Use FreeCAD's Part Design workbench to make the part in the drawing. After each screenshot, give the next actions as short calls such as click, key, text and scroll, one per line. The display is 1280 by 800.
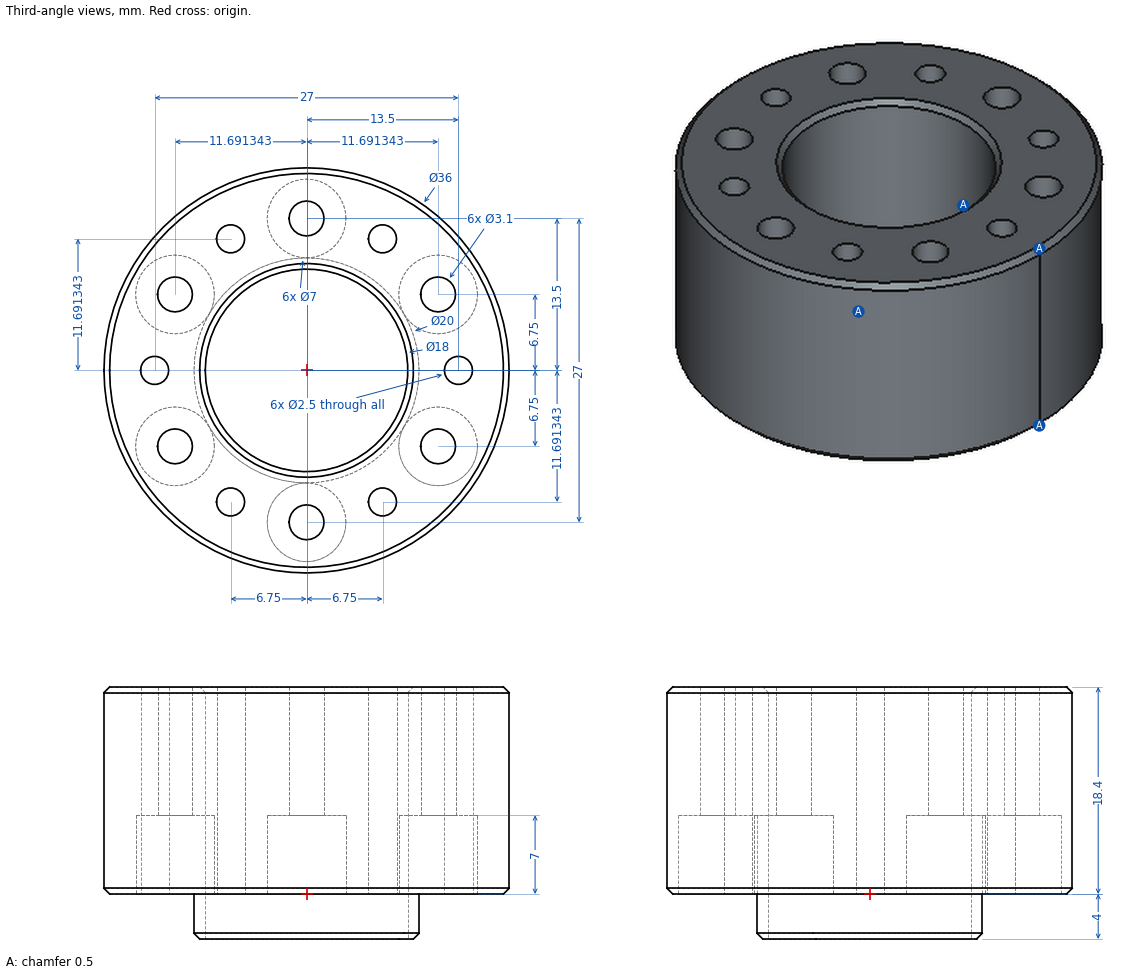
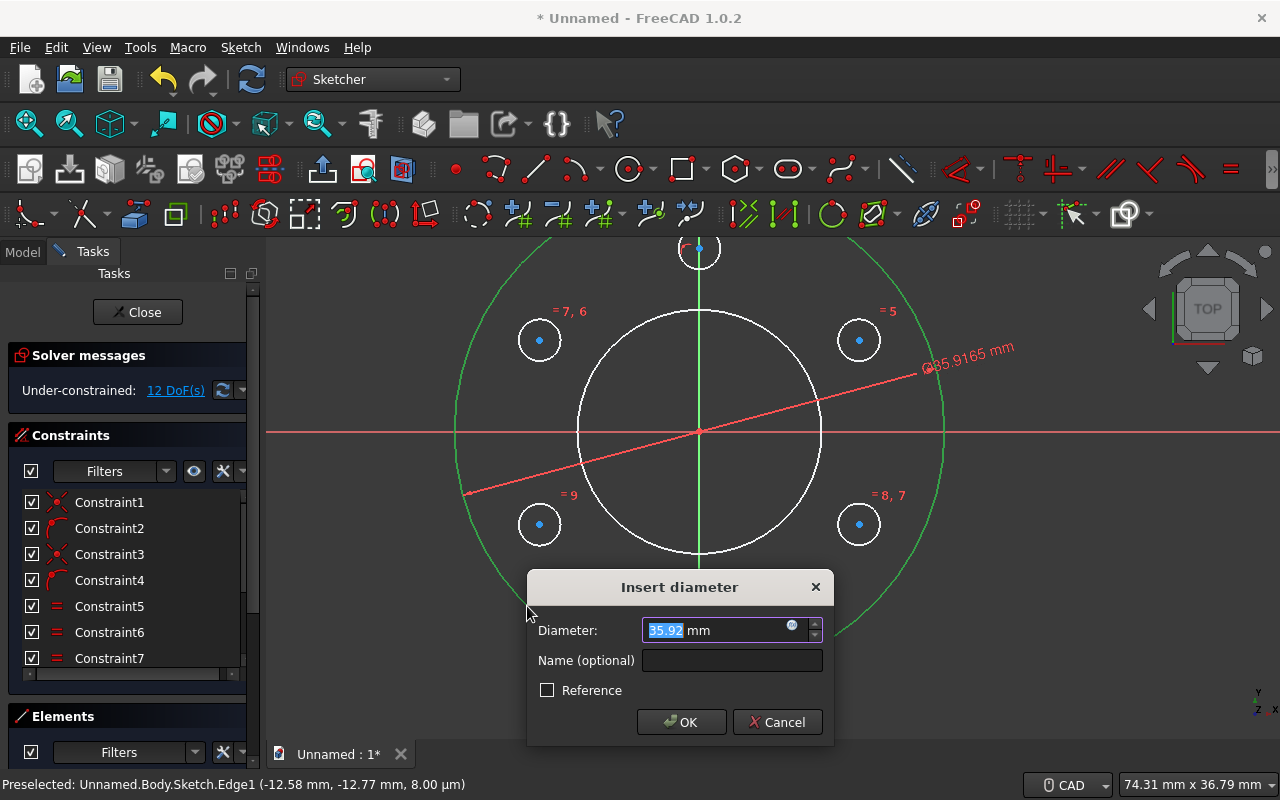
text(36)
key(Return)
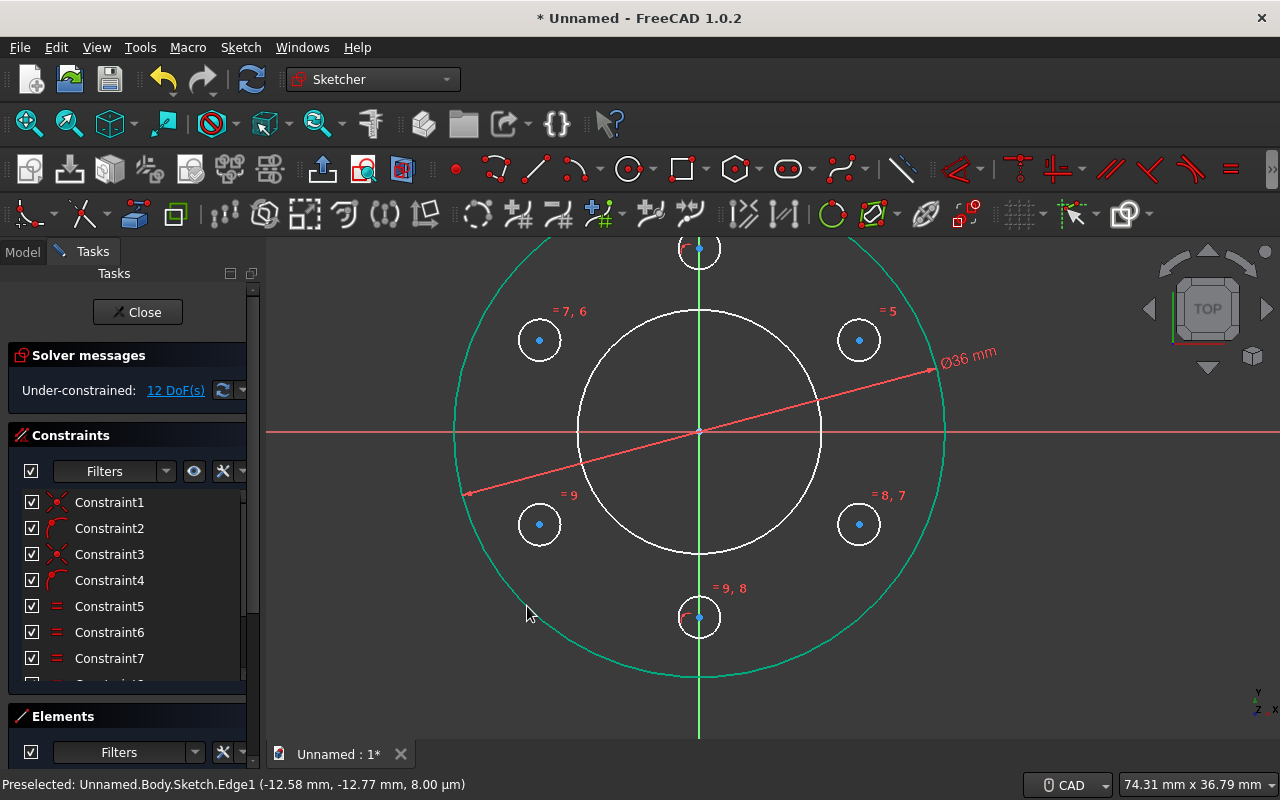
click(874, 325)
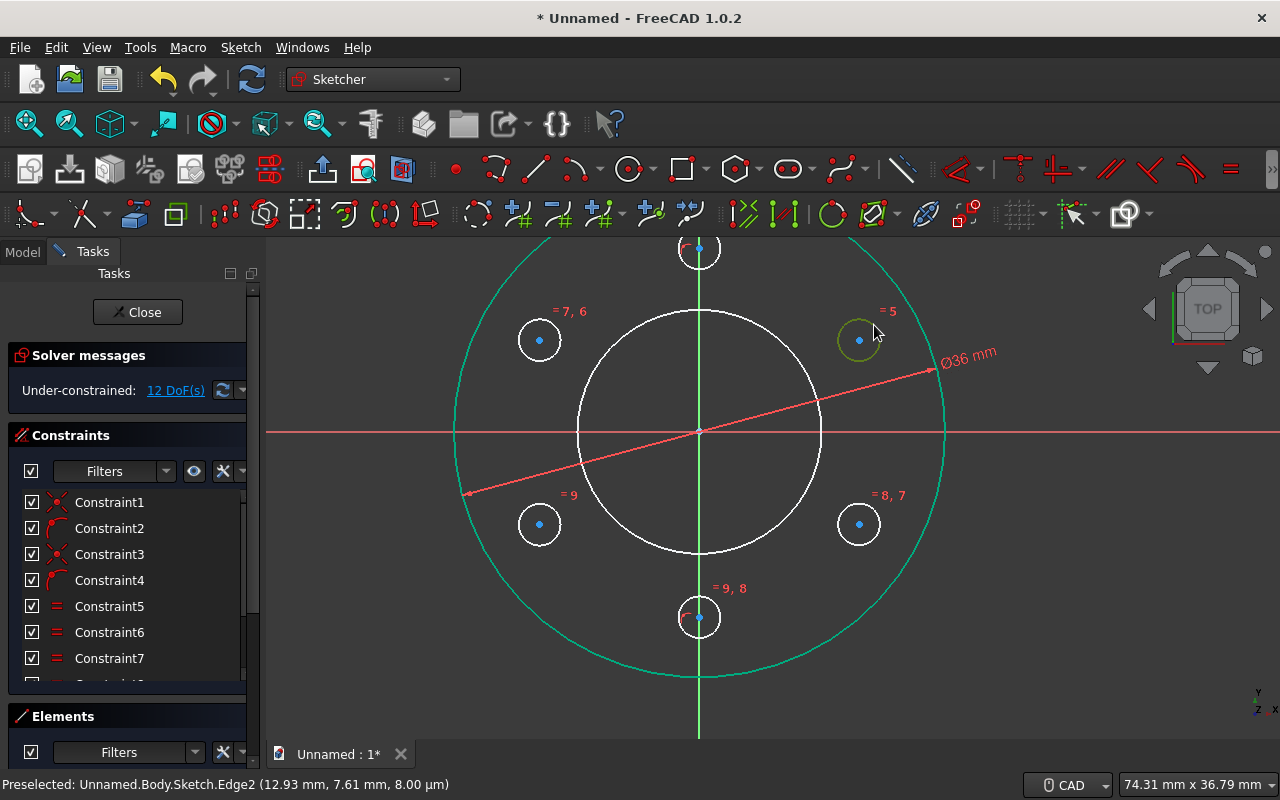
click(982, 170)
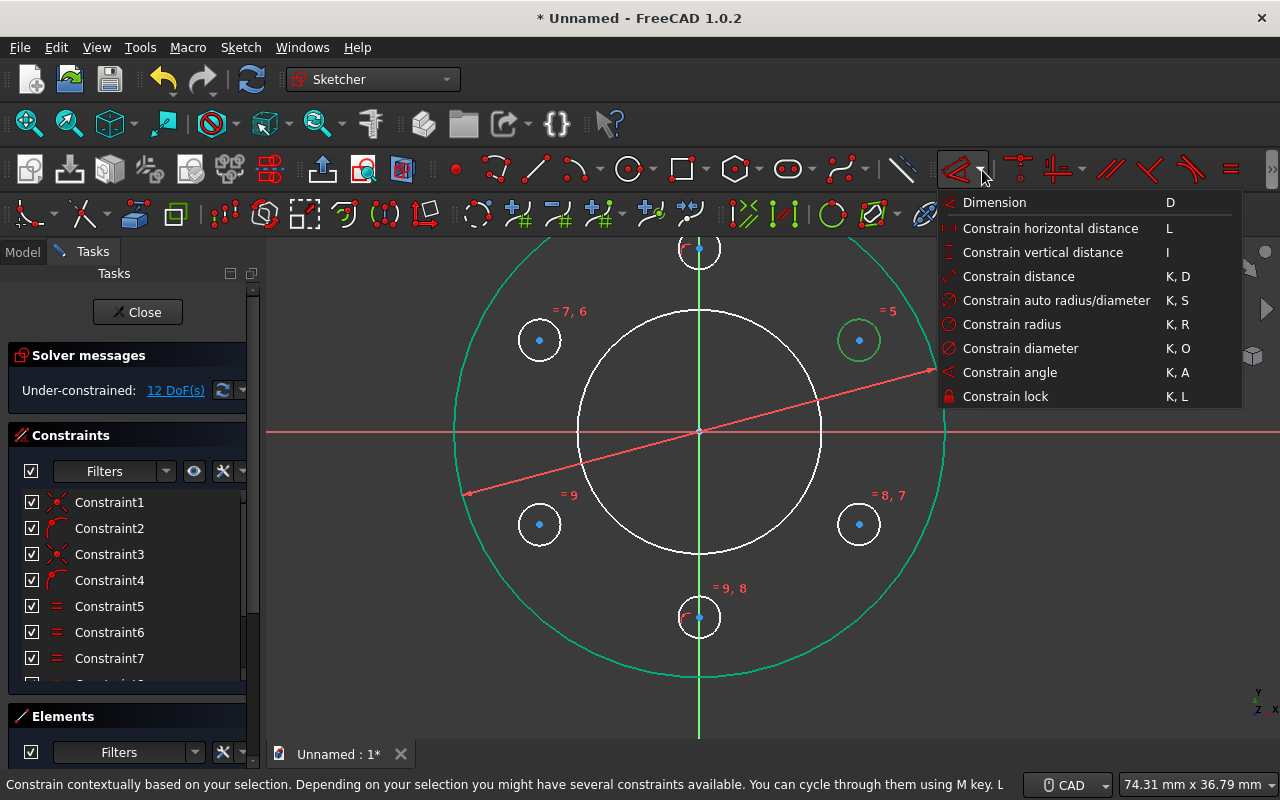
click(1090, 348)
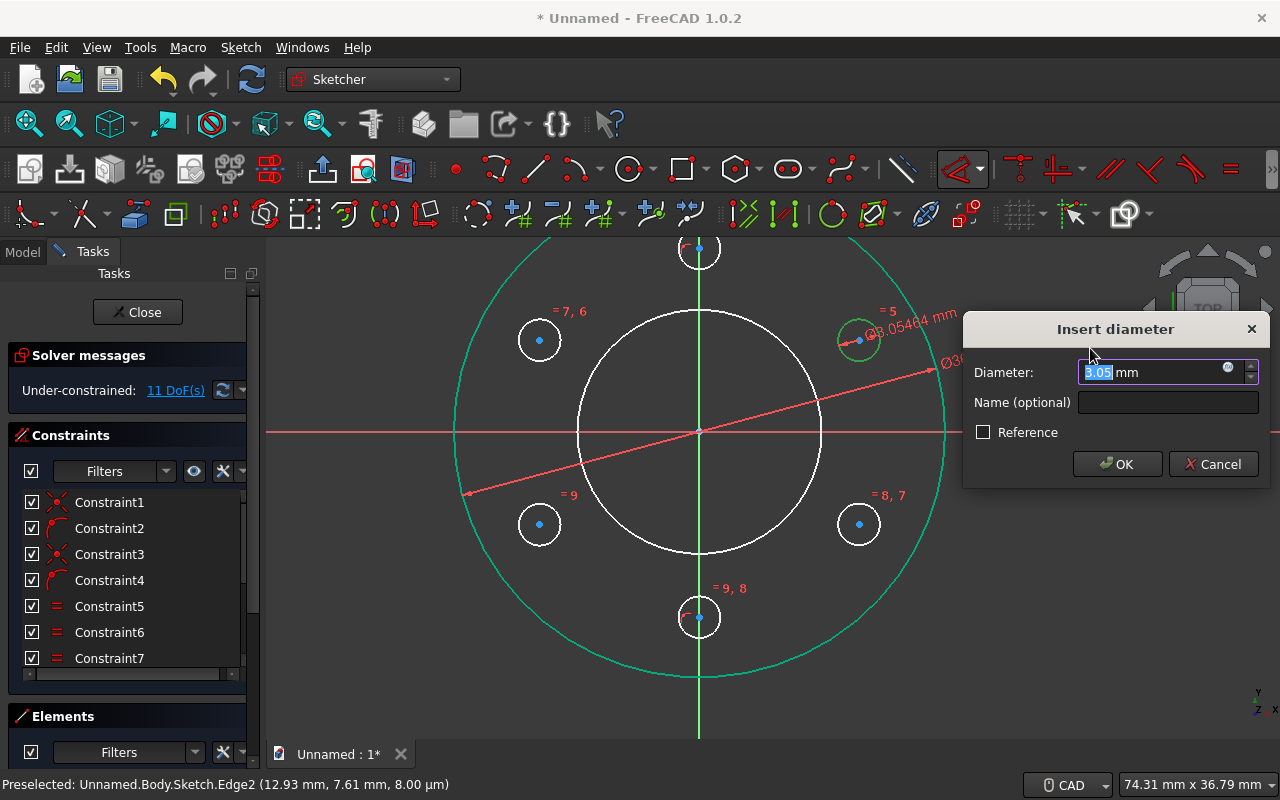
text(3.1)
key(Return)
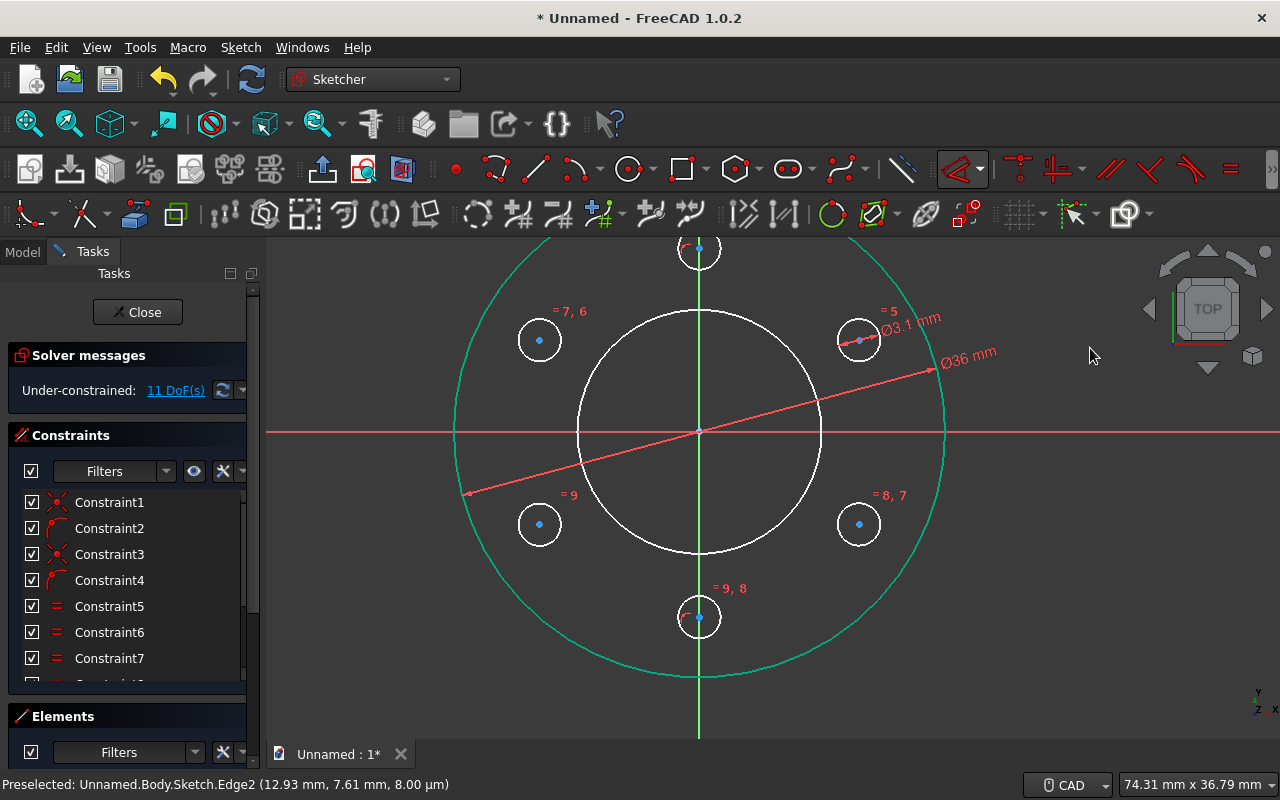
click(785, 345)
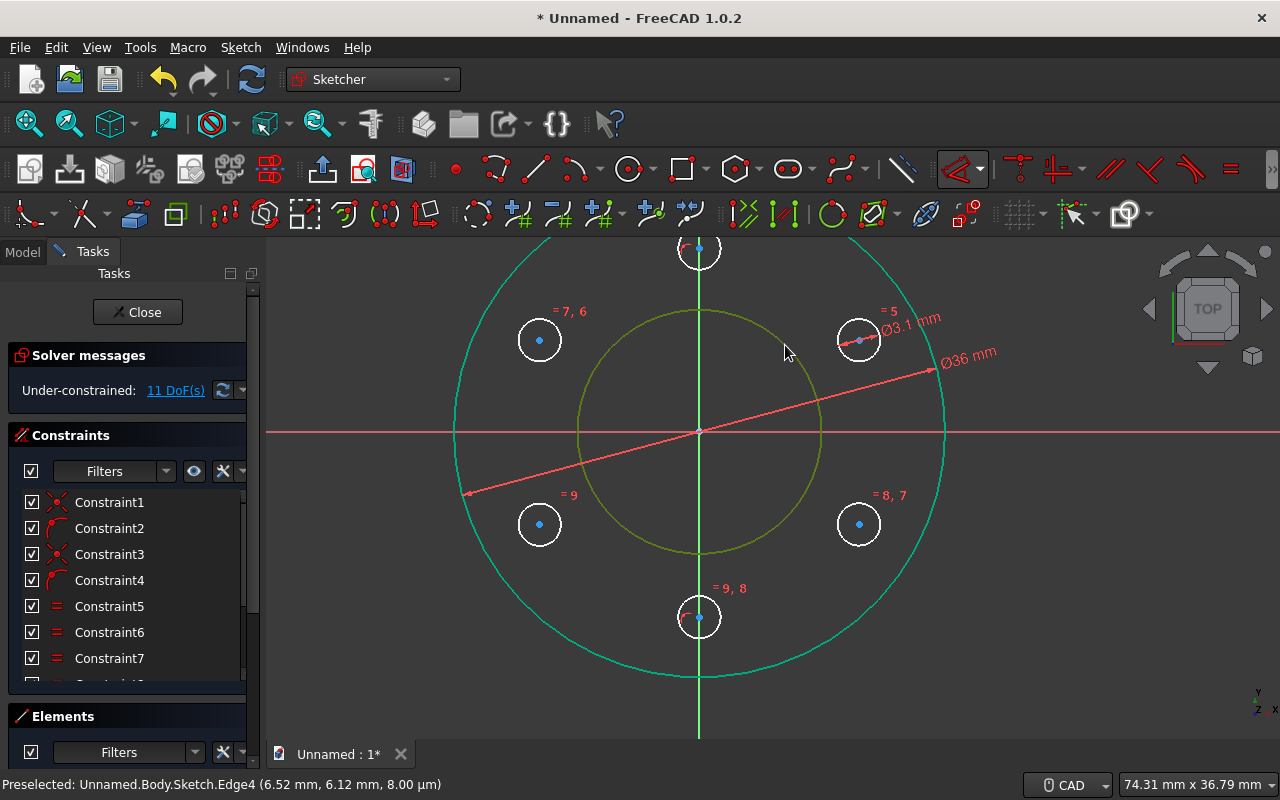
key(k)
key(o)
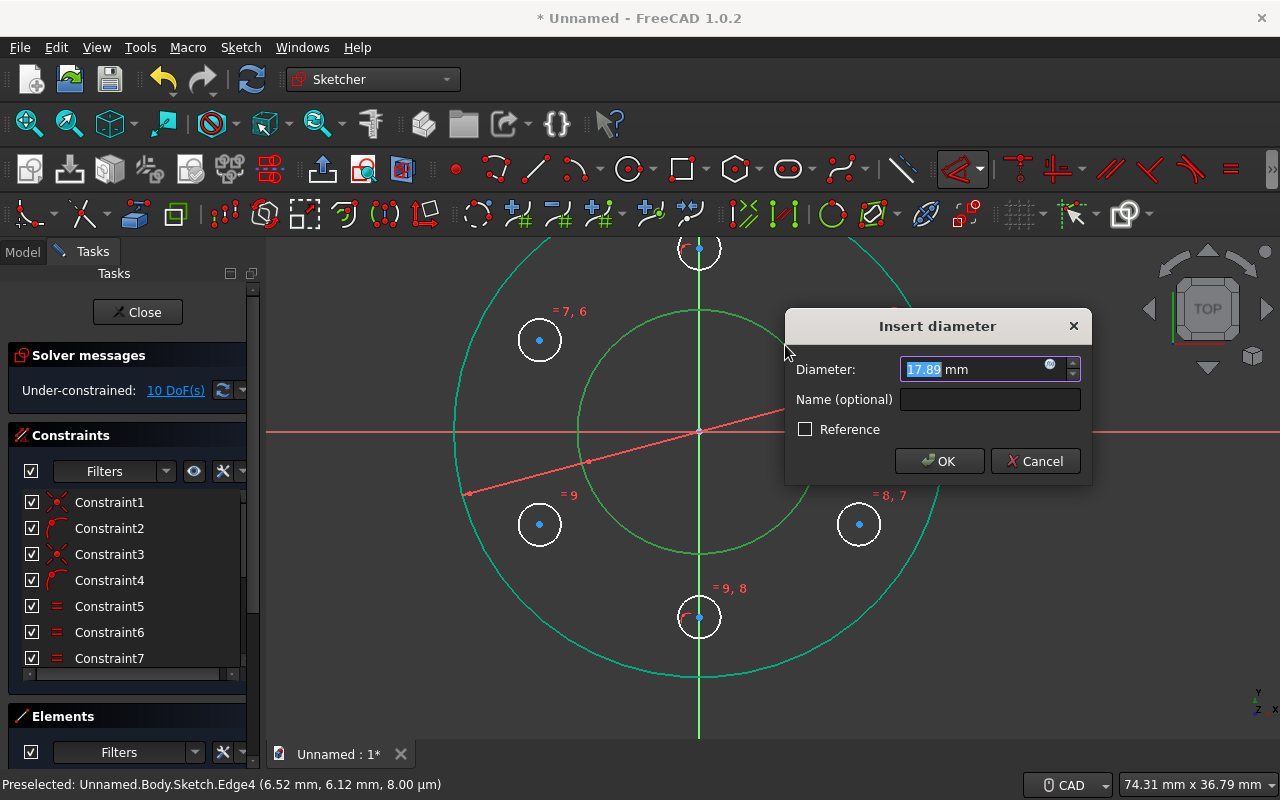
text(18)
key(Return)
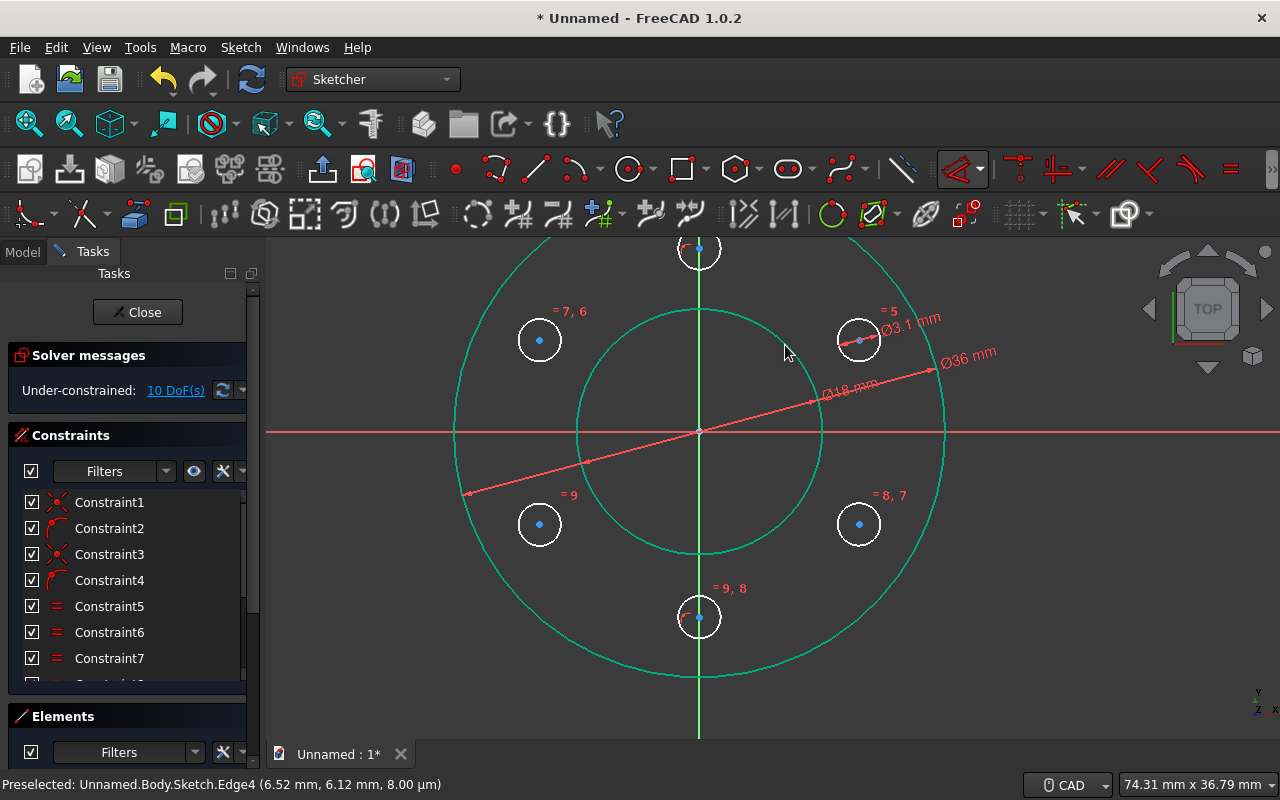
scroll(715, 602, down, 2)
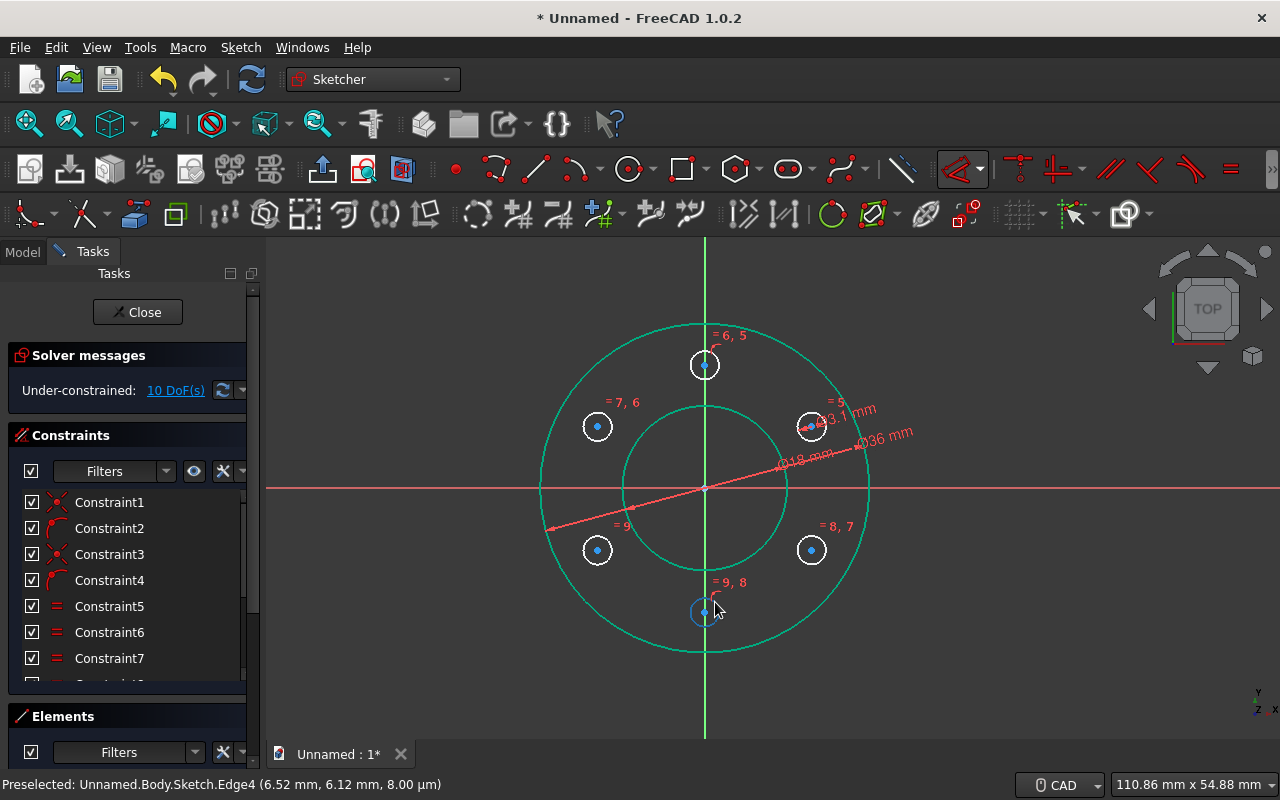
click(705, 365)